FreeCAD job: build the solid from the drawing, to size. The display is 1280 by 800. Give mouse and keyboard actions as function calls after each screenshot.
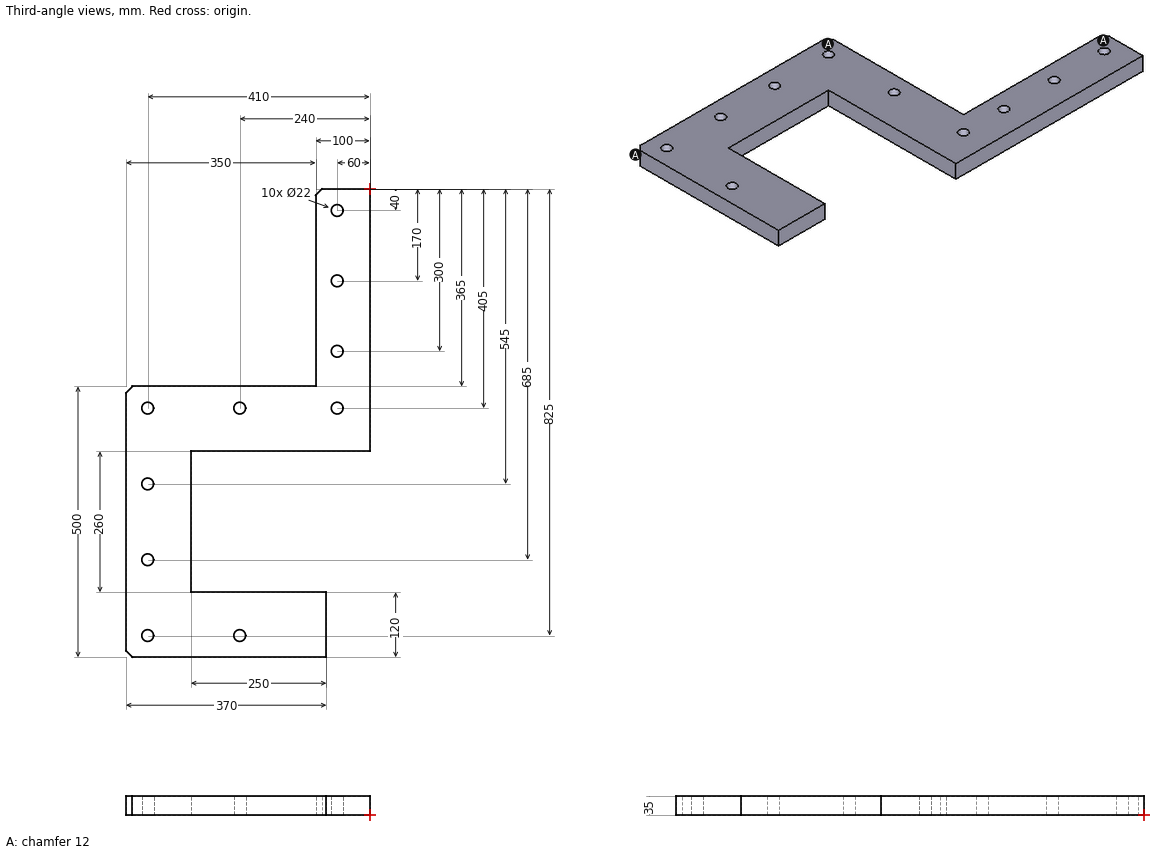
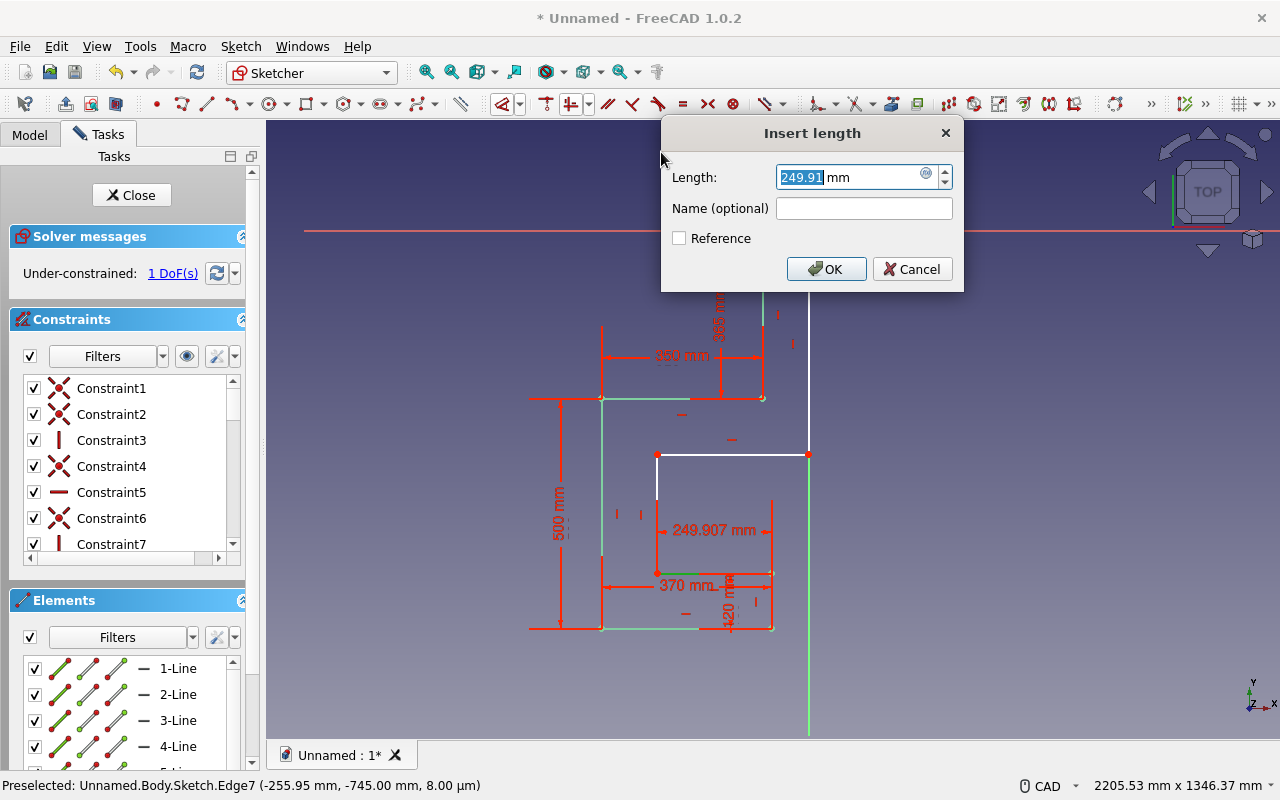
text(250)
key(Return)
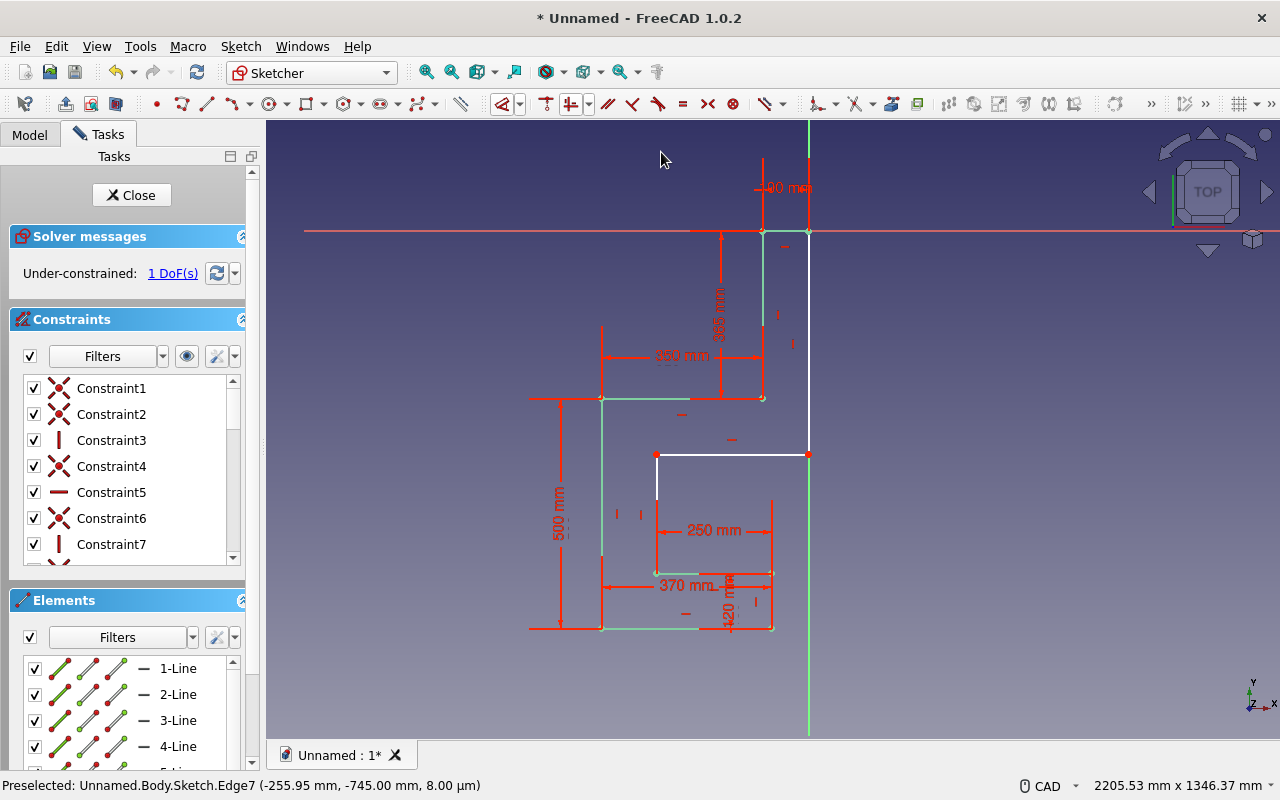
click(657, 538)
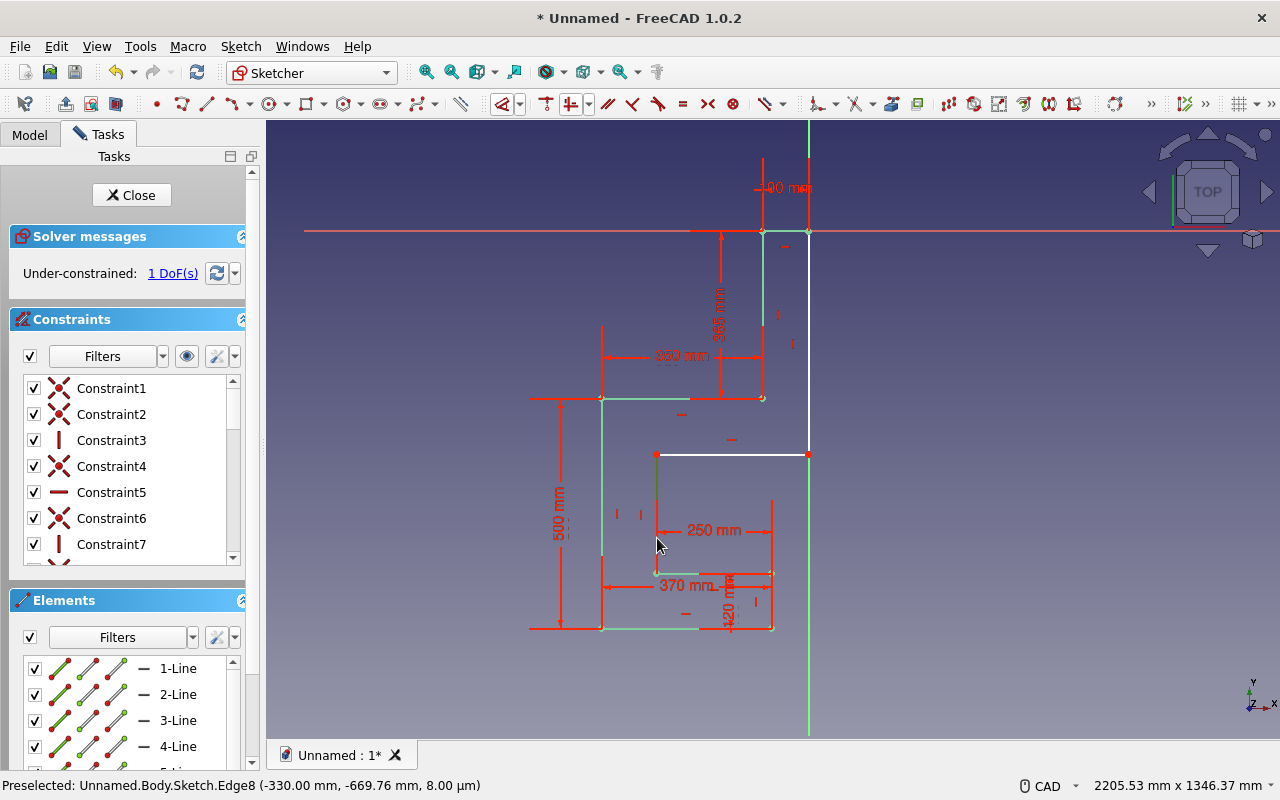
click(520, 104)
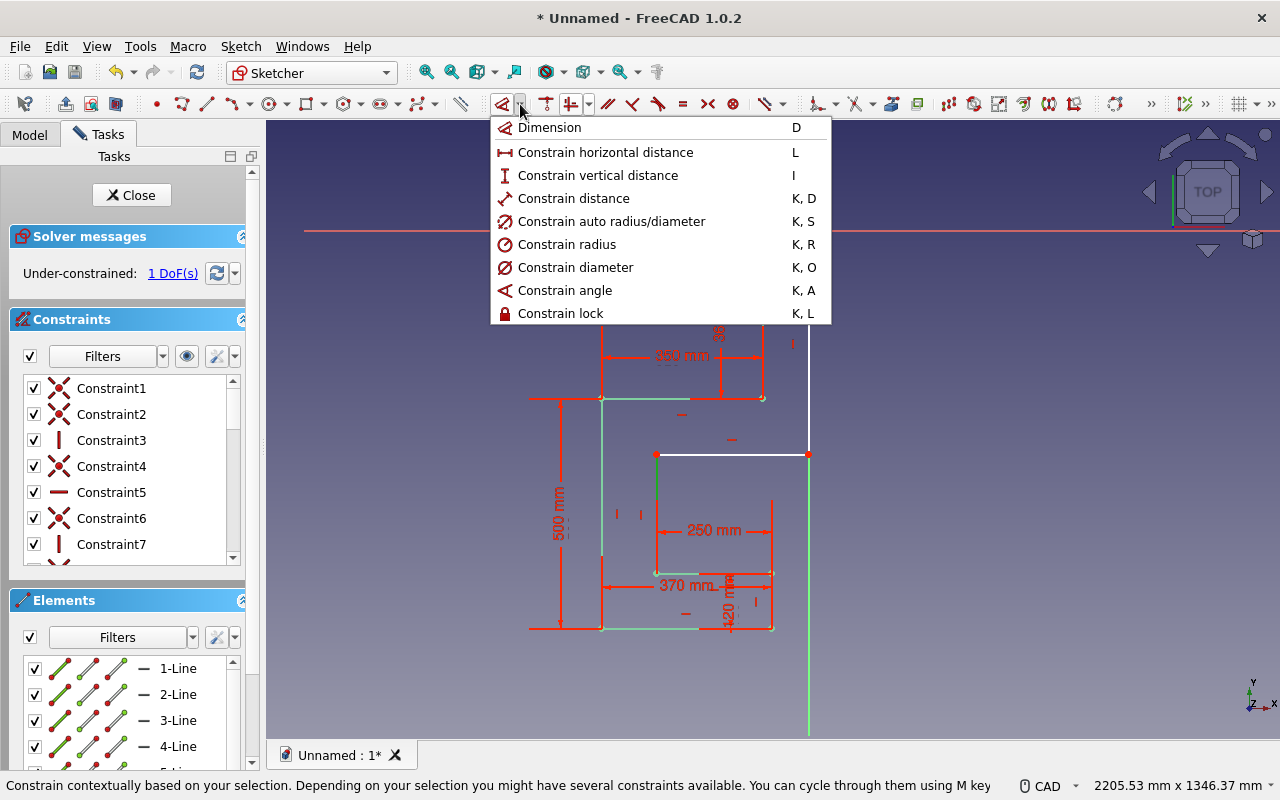
click(661, 176)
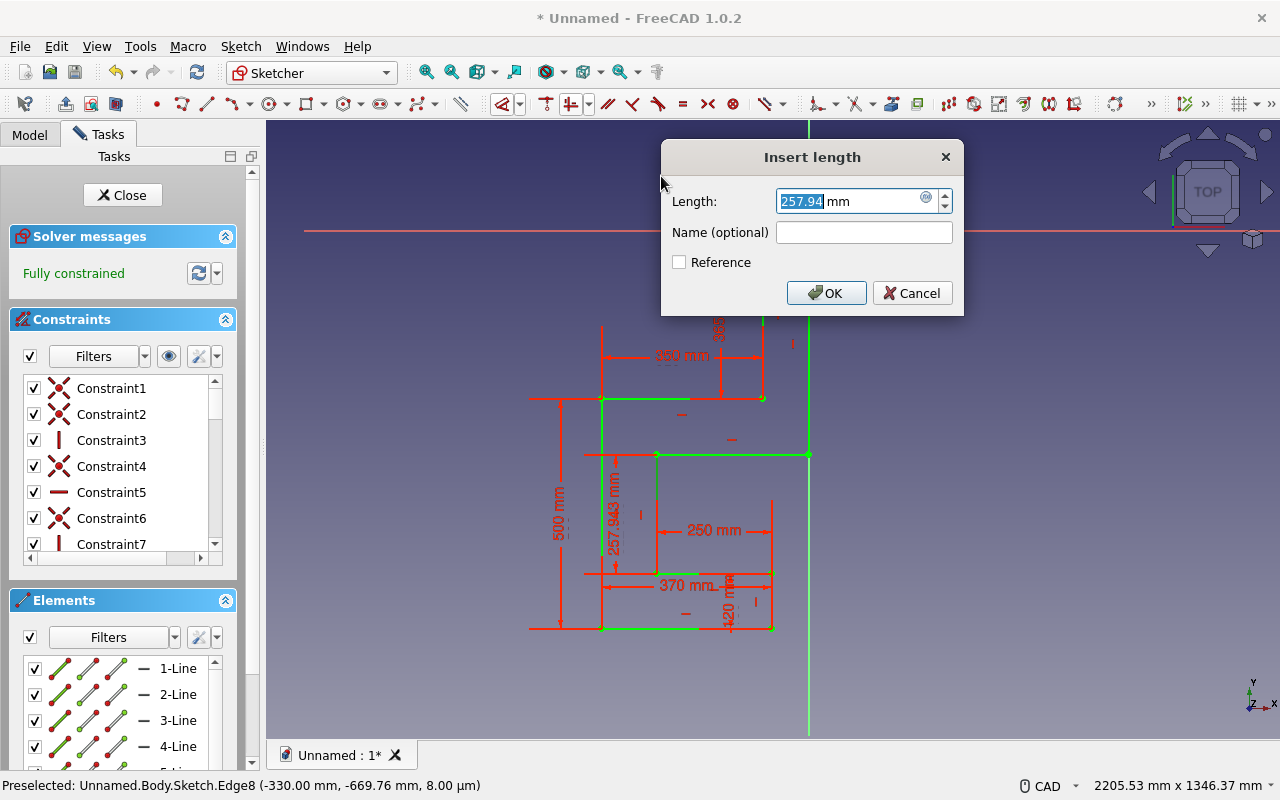
text(260)
key(Return)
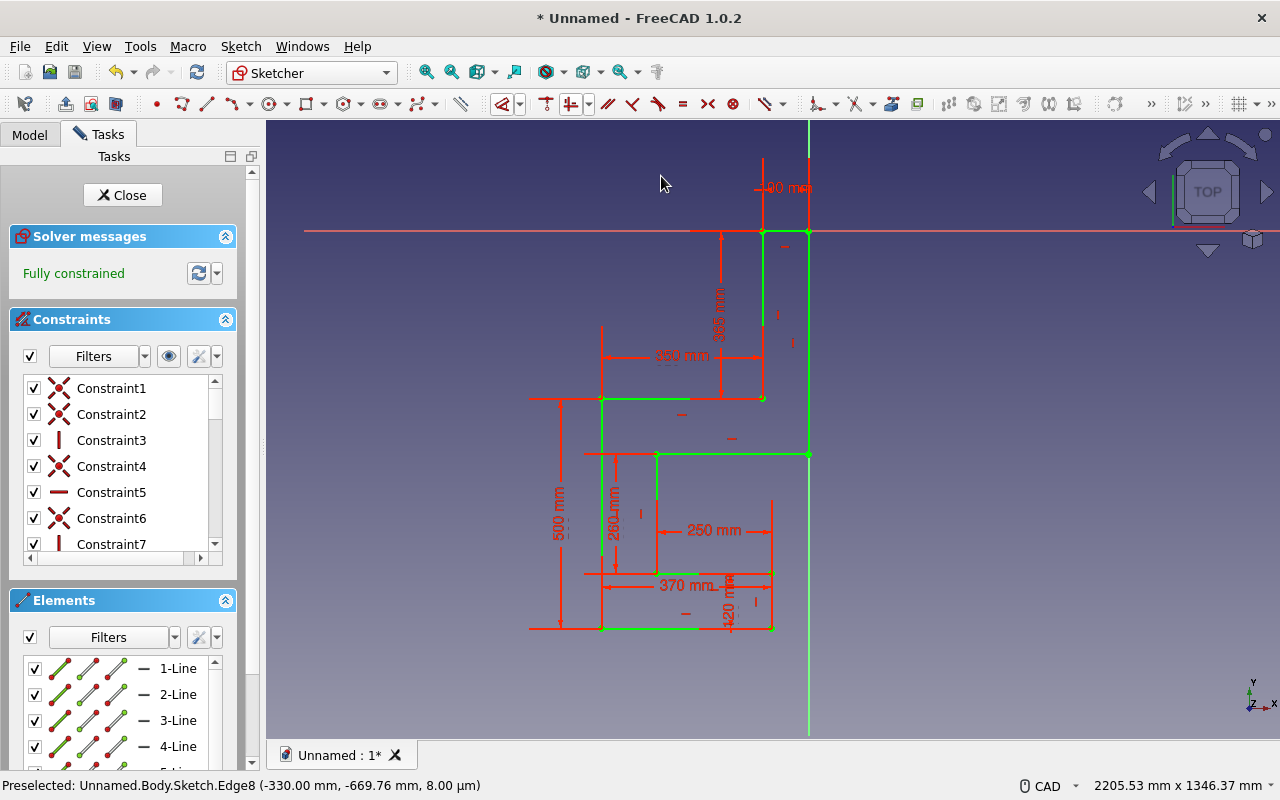
click(123, 195)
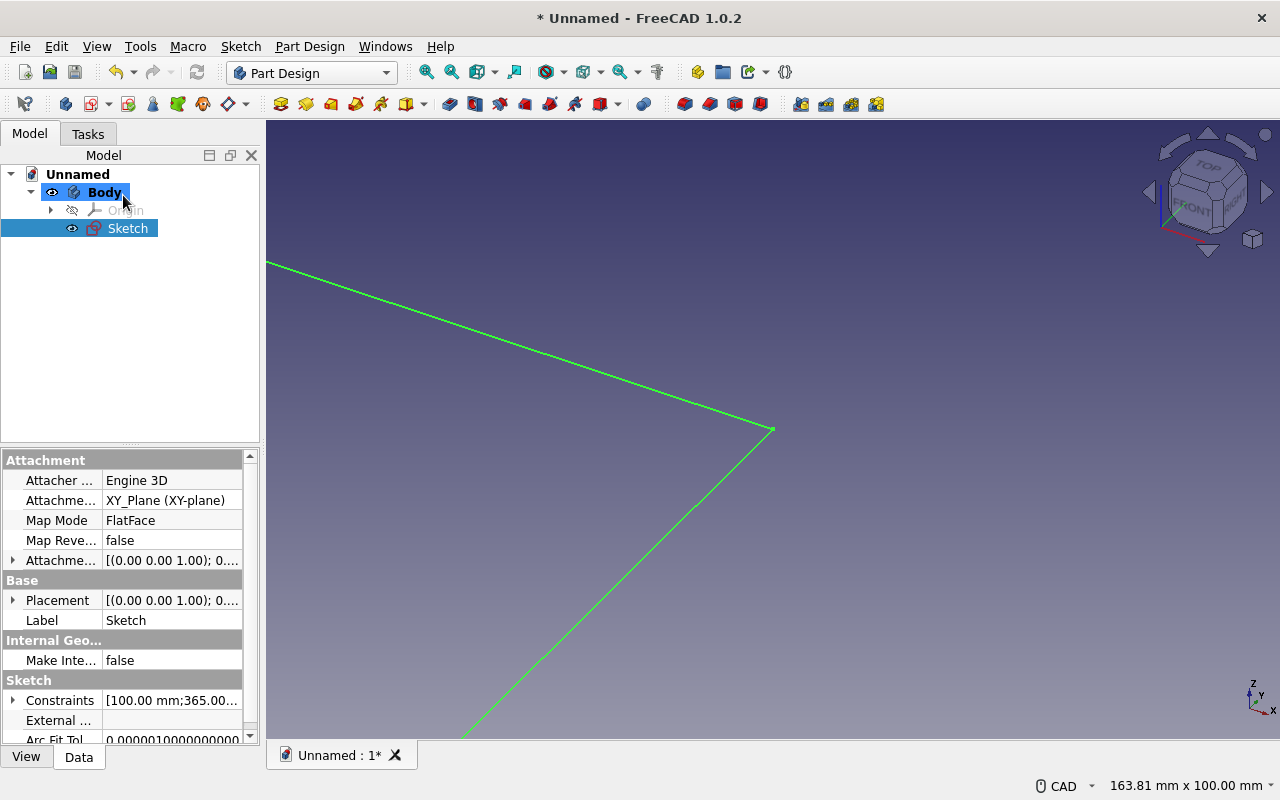
click(281, 104)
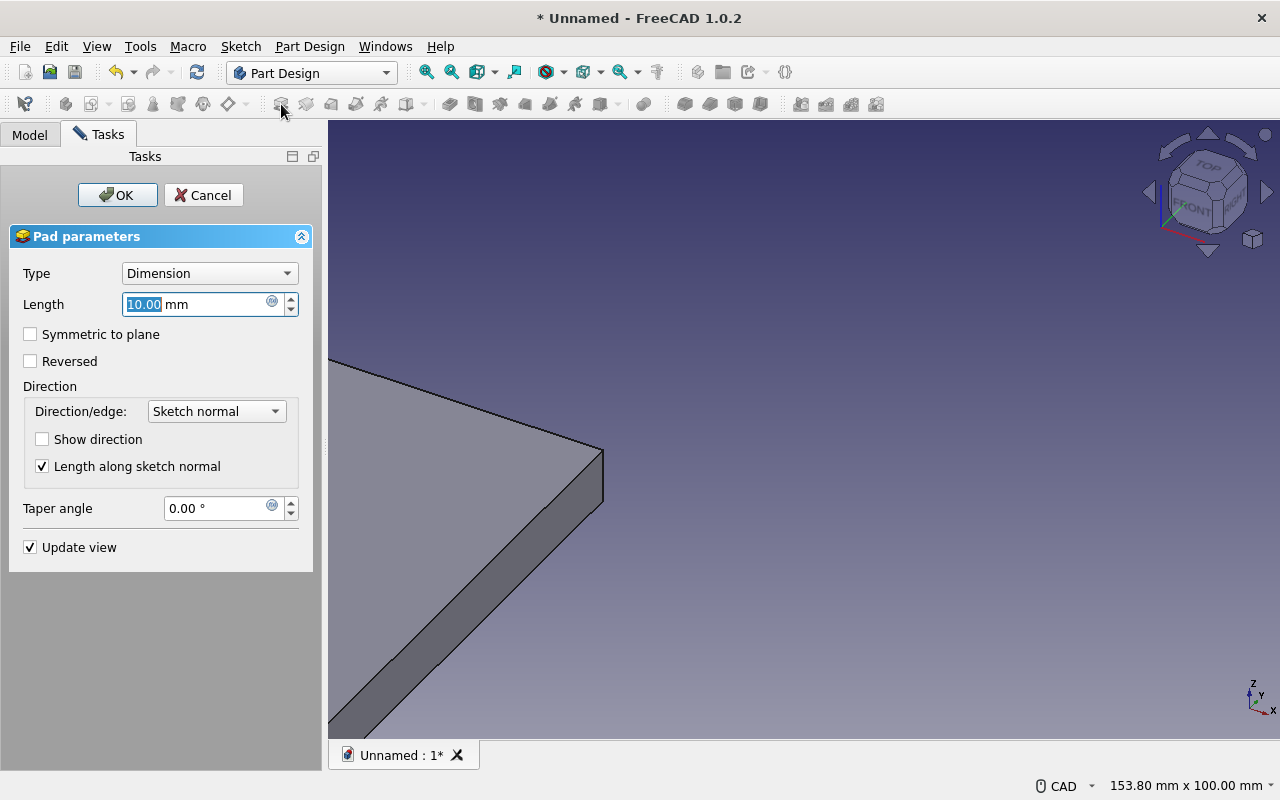
text(35)
key(Tab)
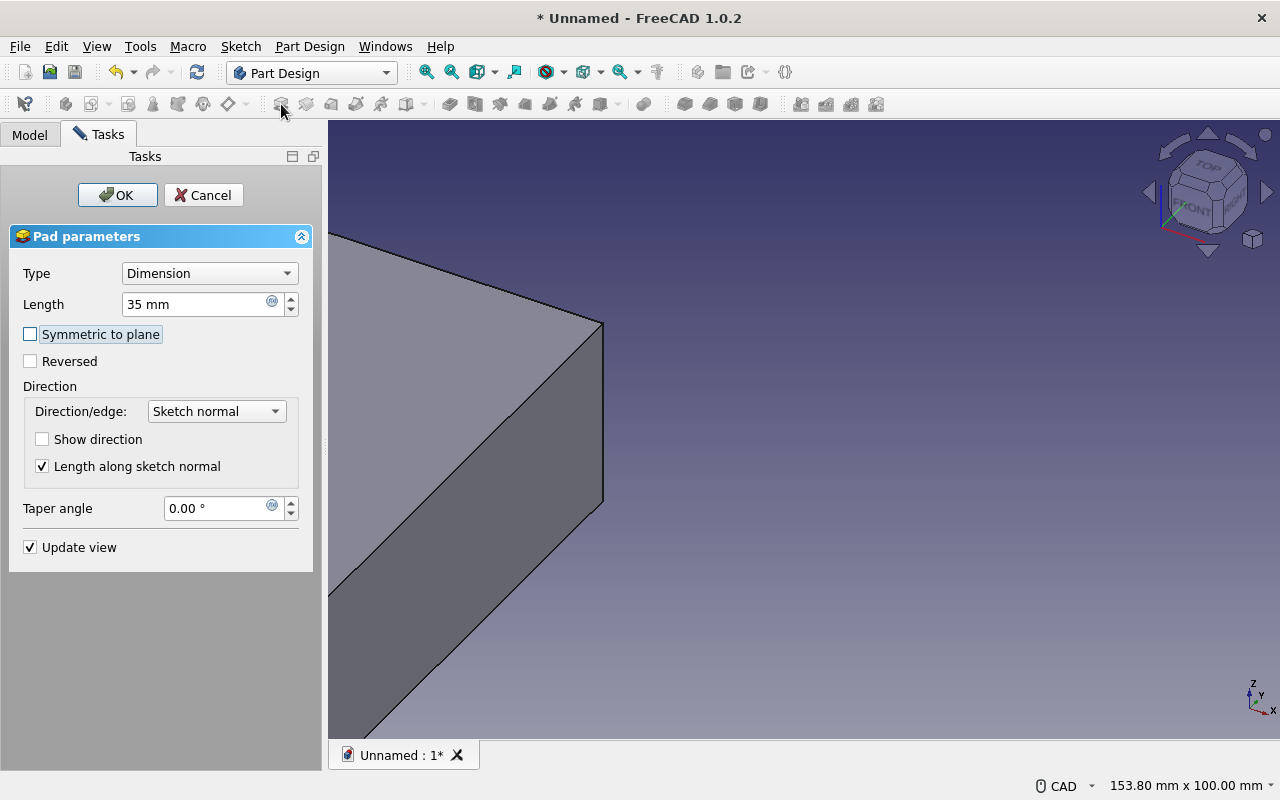
click(118, 195)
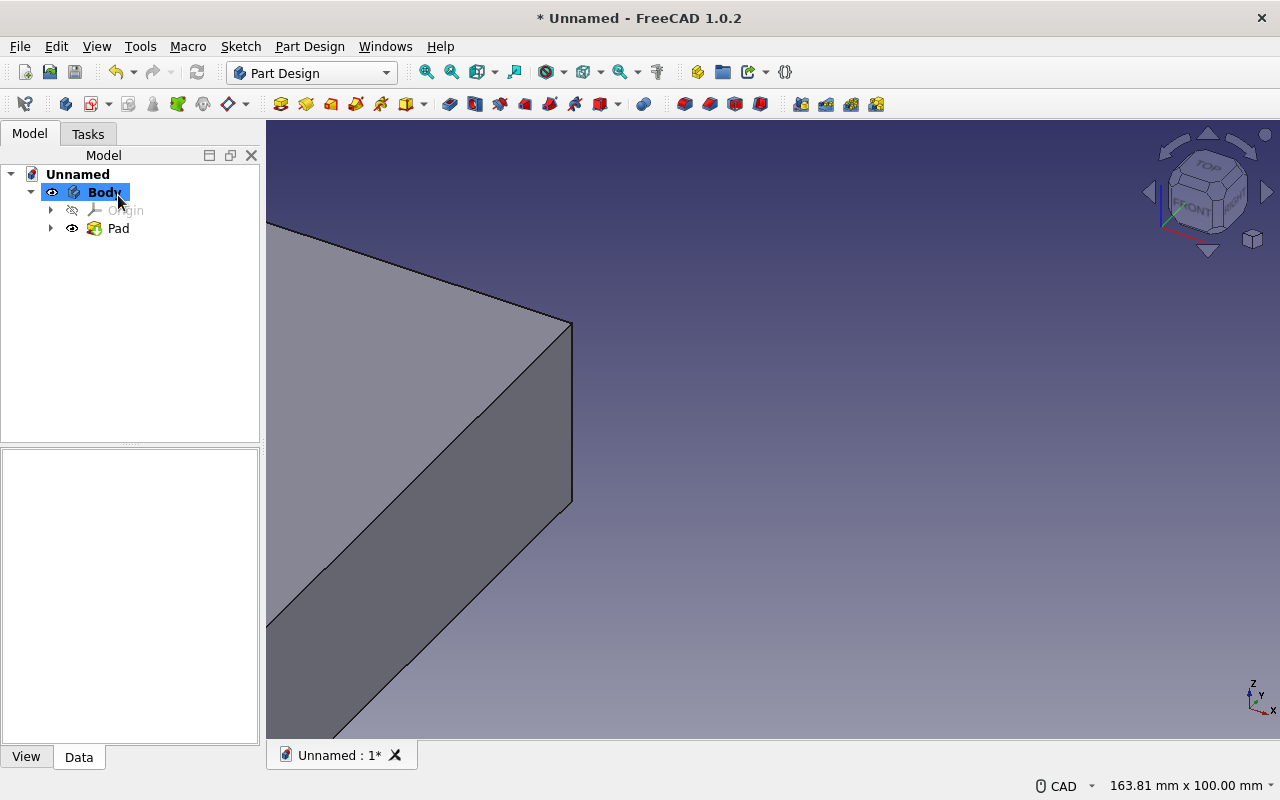
click(427, 72)